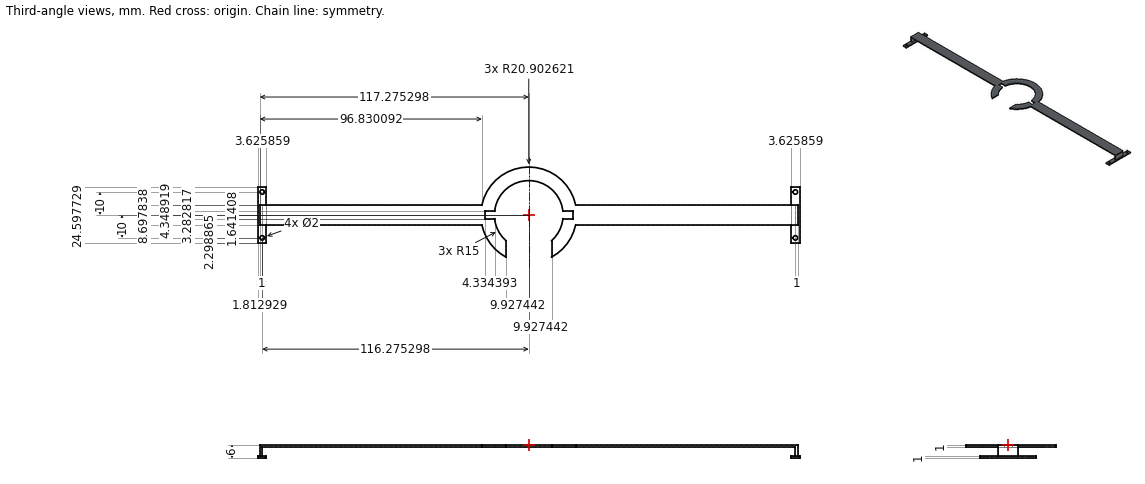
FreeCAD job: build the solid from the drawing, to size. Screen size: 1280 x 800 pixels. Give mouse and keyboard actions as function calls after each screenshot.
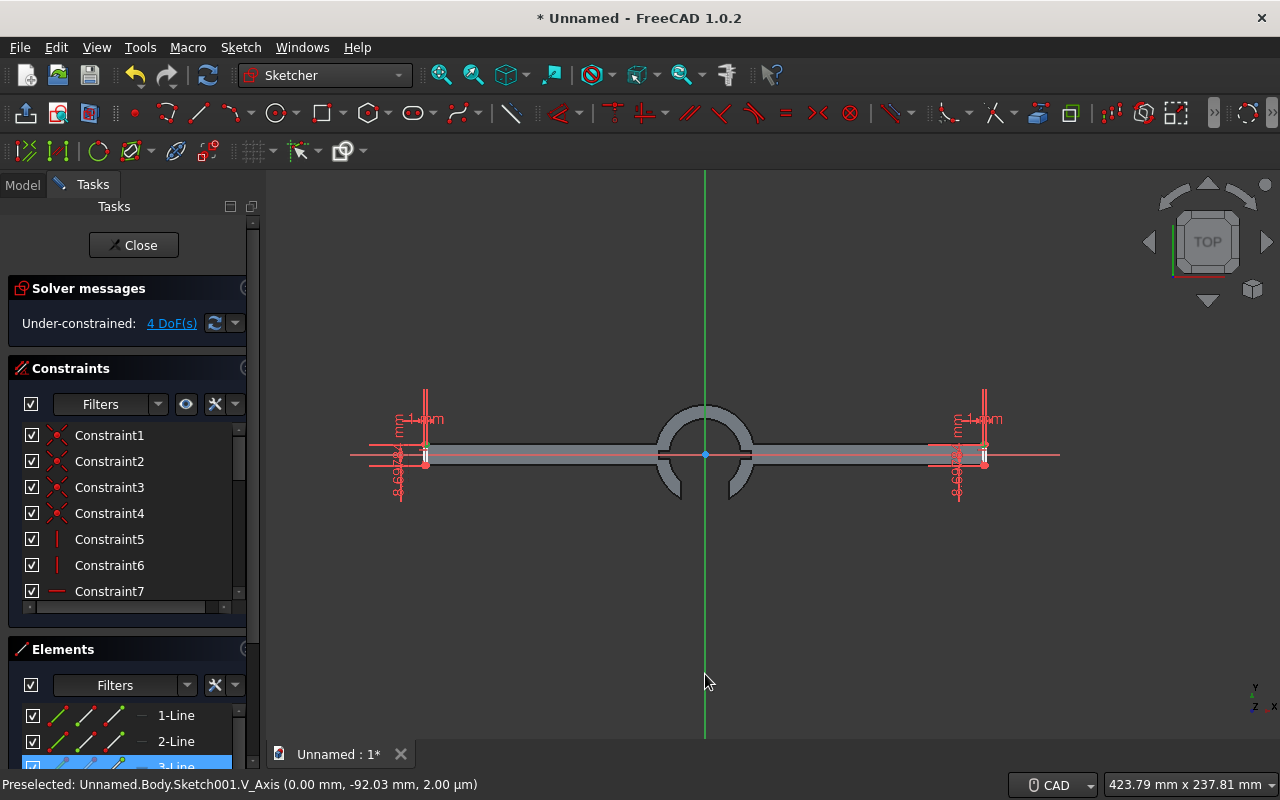
click(818, 114)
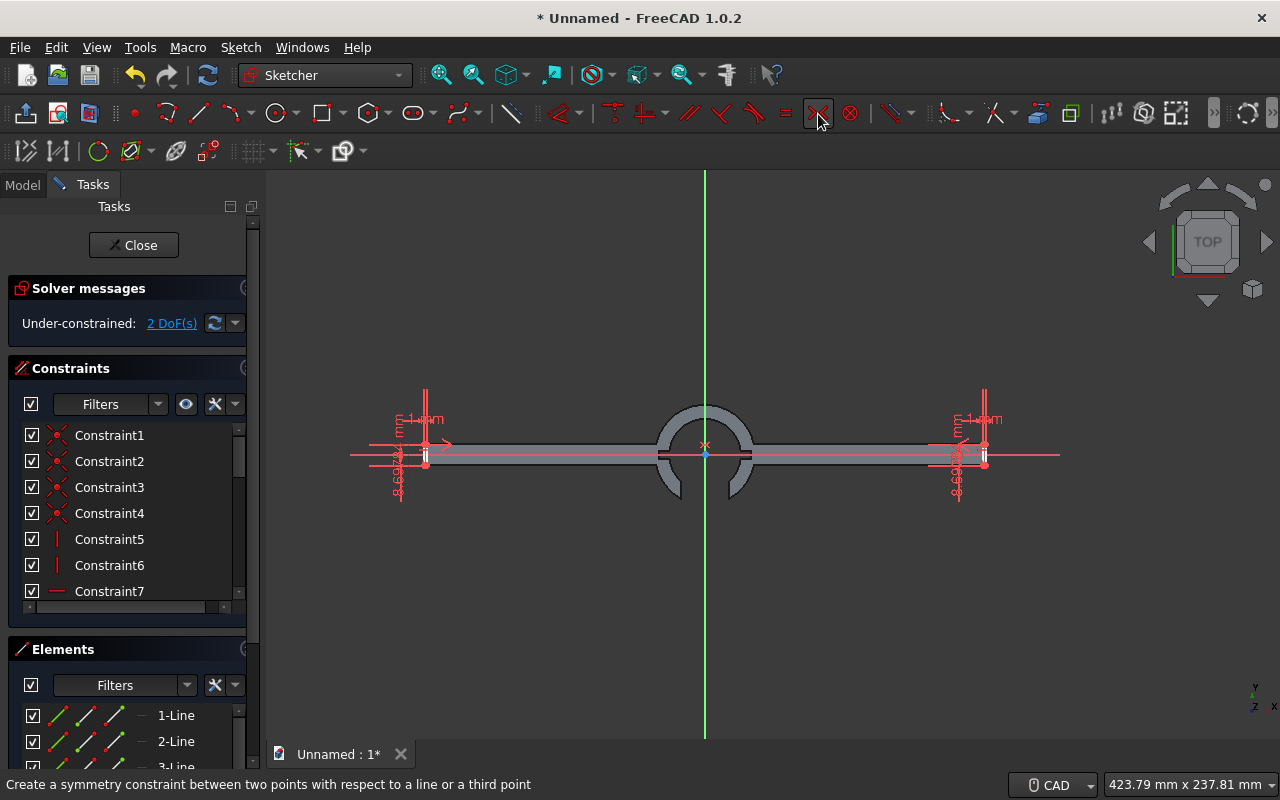
click(558, 114)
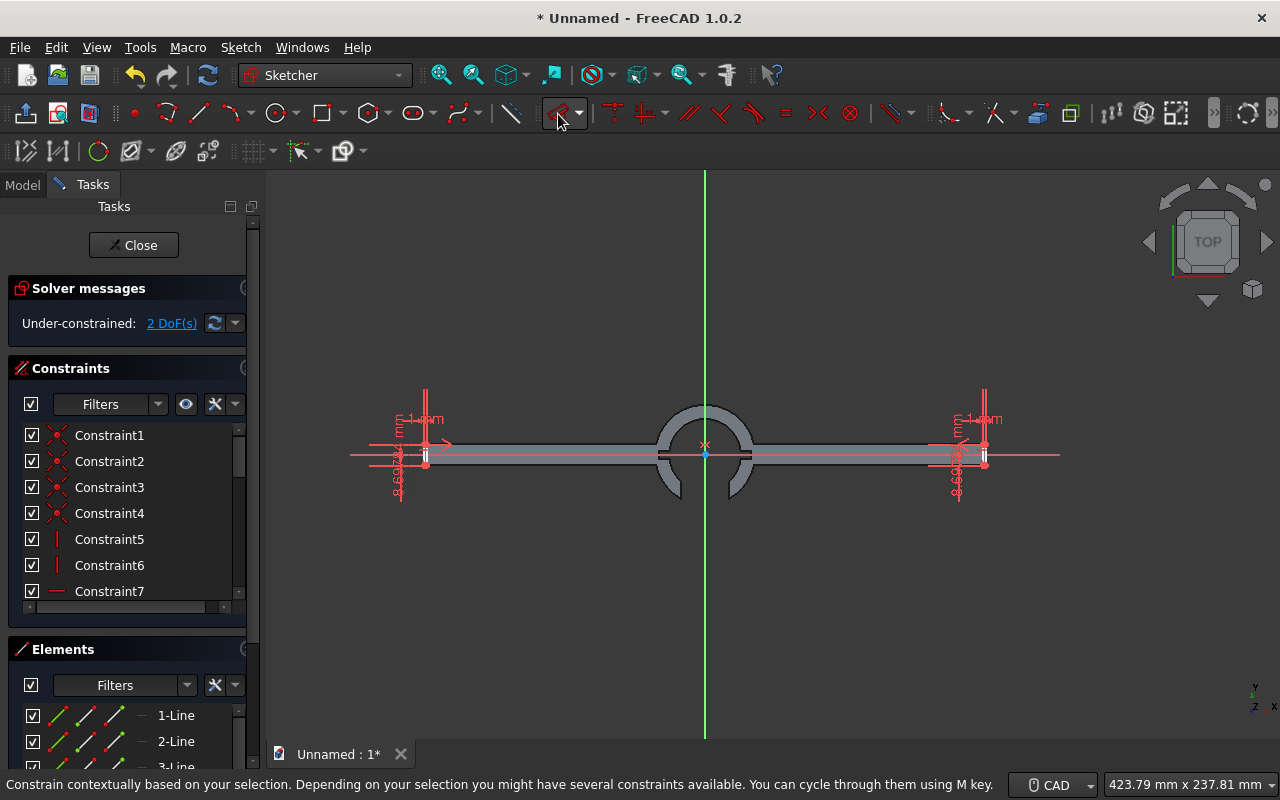
scroll(424, 445, up, 9)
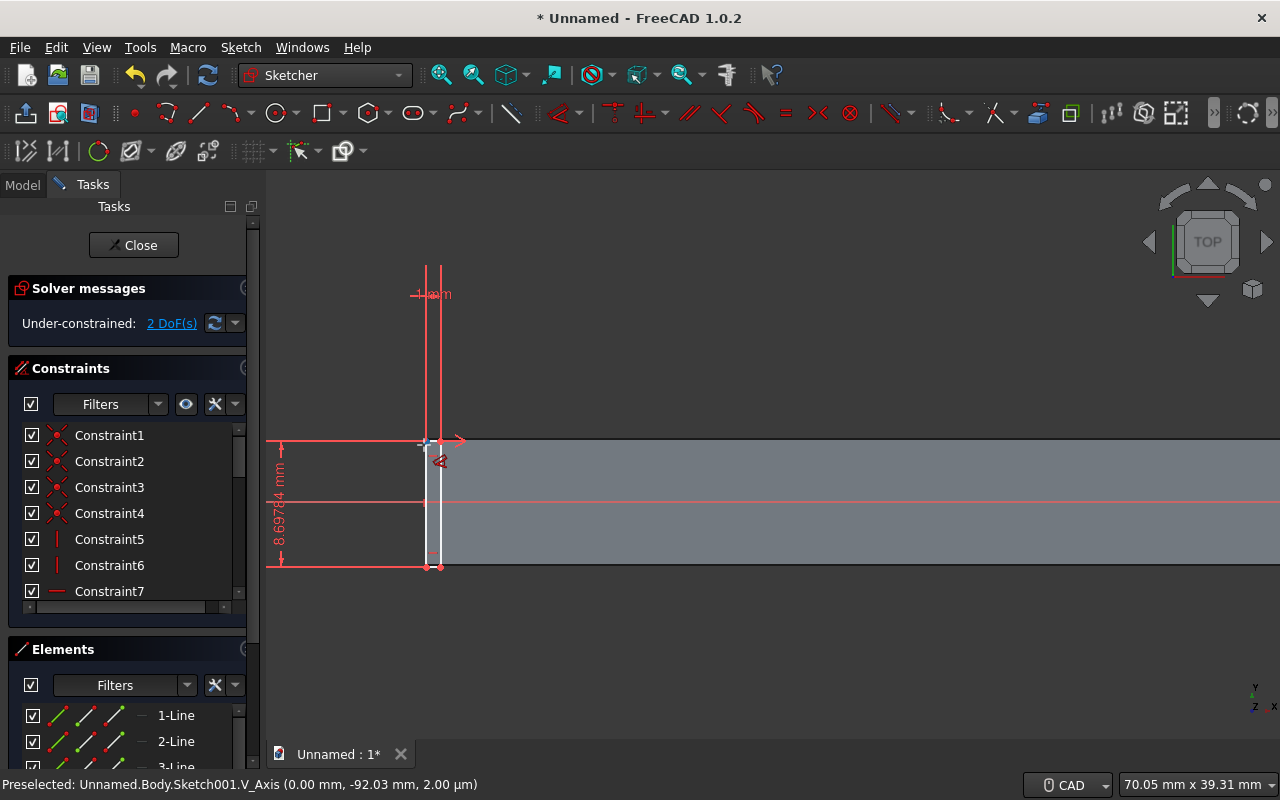
click(426, 441)
click(392, 471)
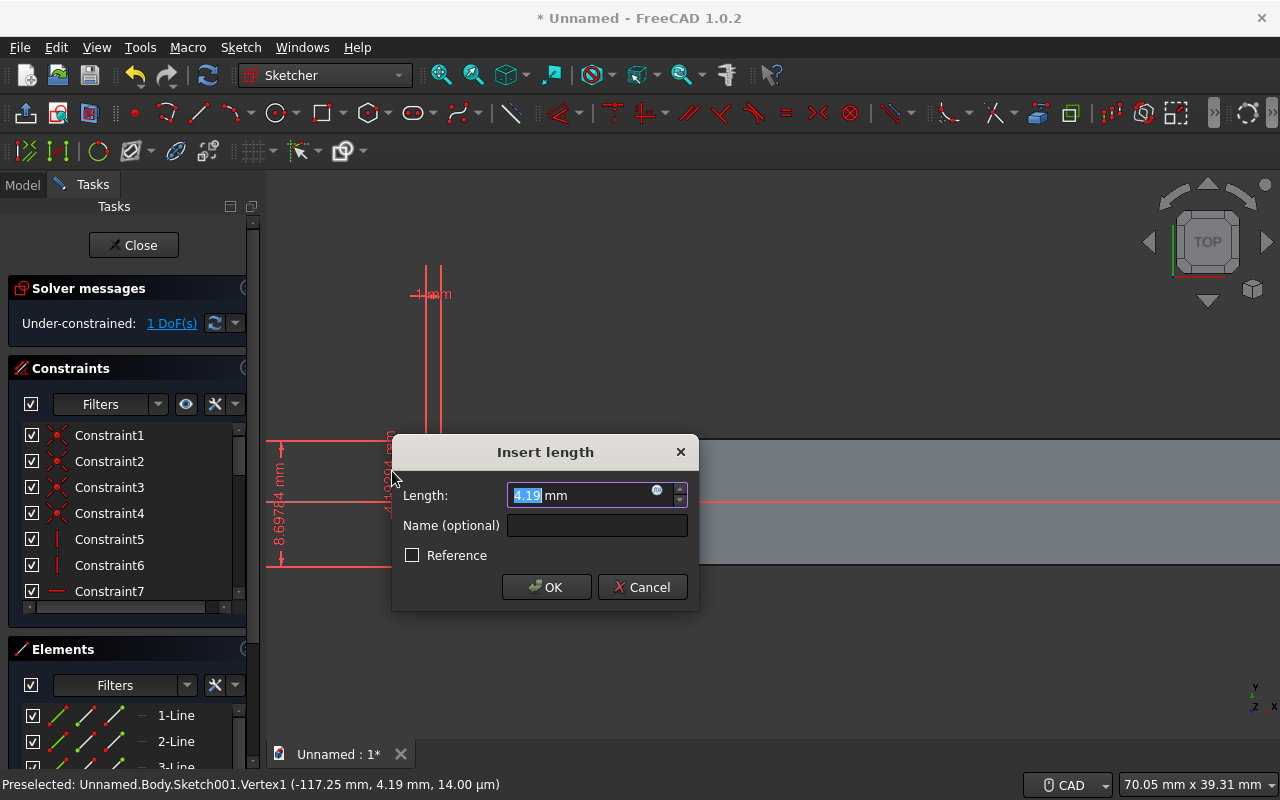
text(4.348919)
key(Return)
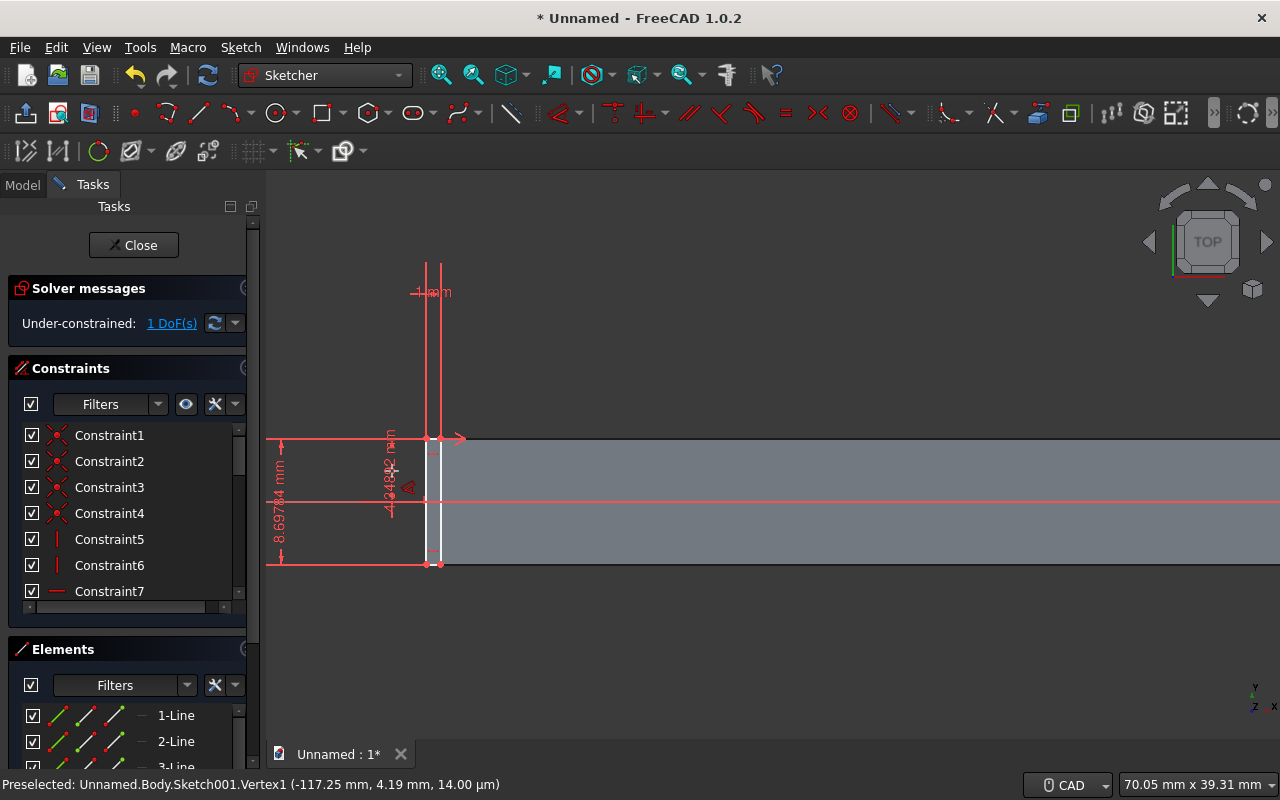
click(426, 439)
click(771, 405)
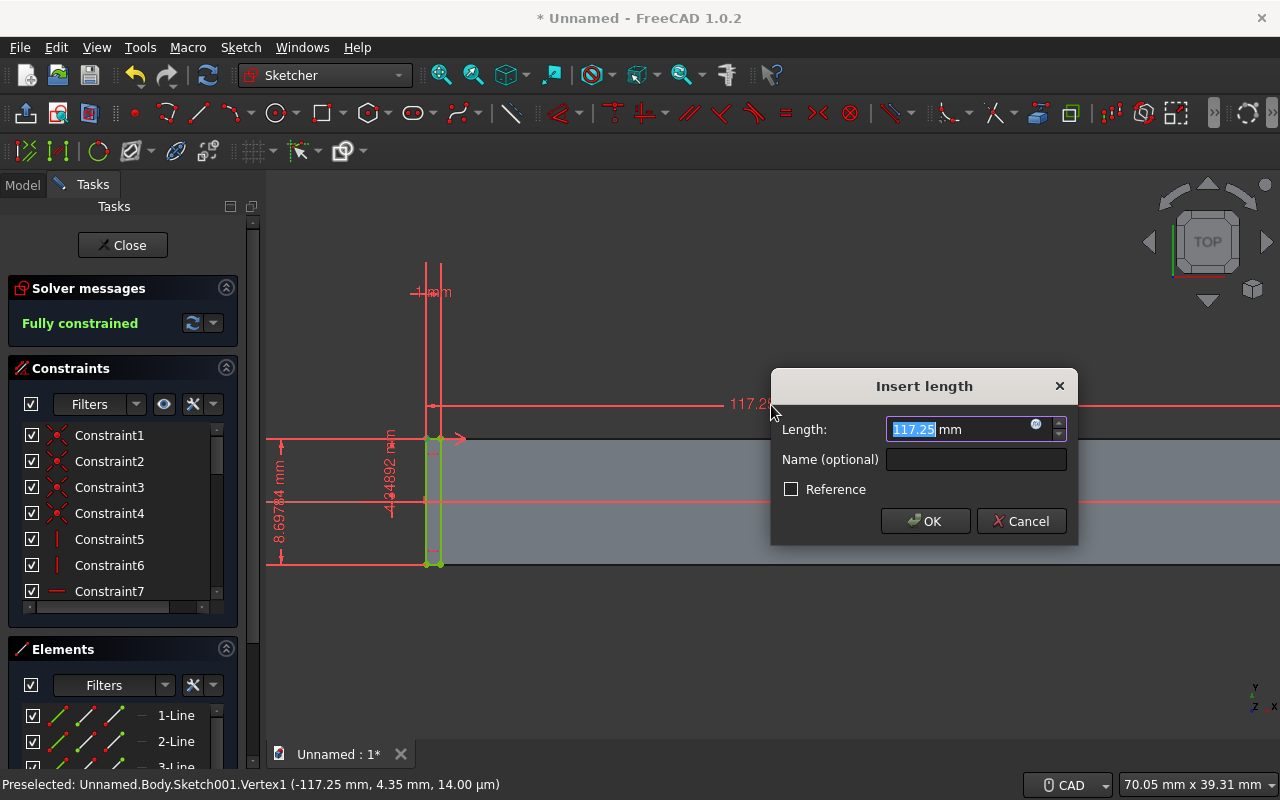
text(117.275298)
key(Return)
key(Escape)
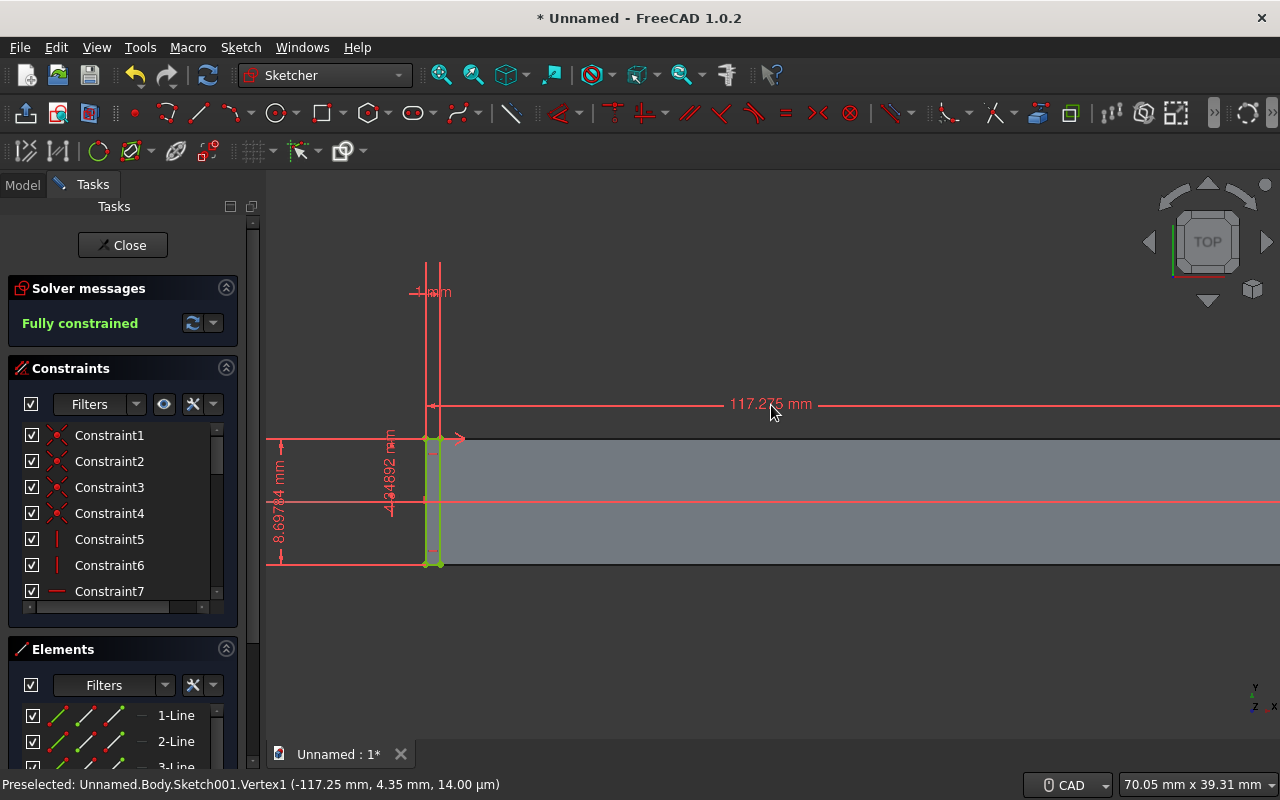
click(123, 245)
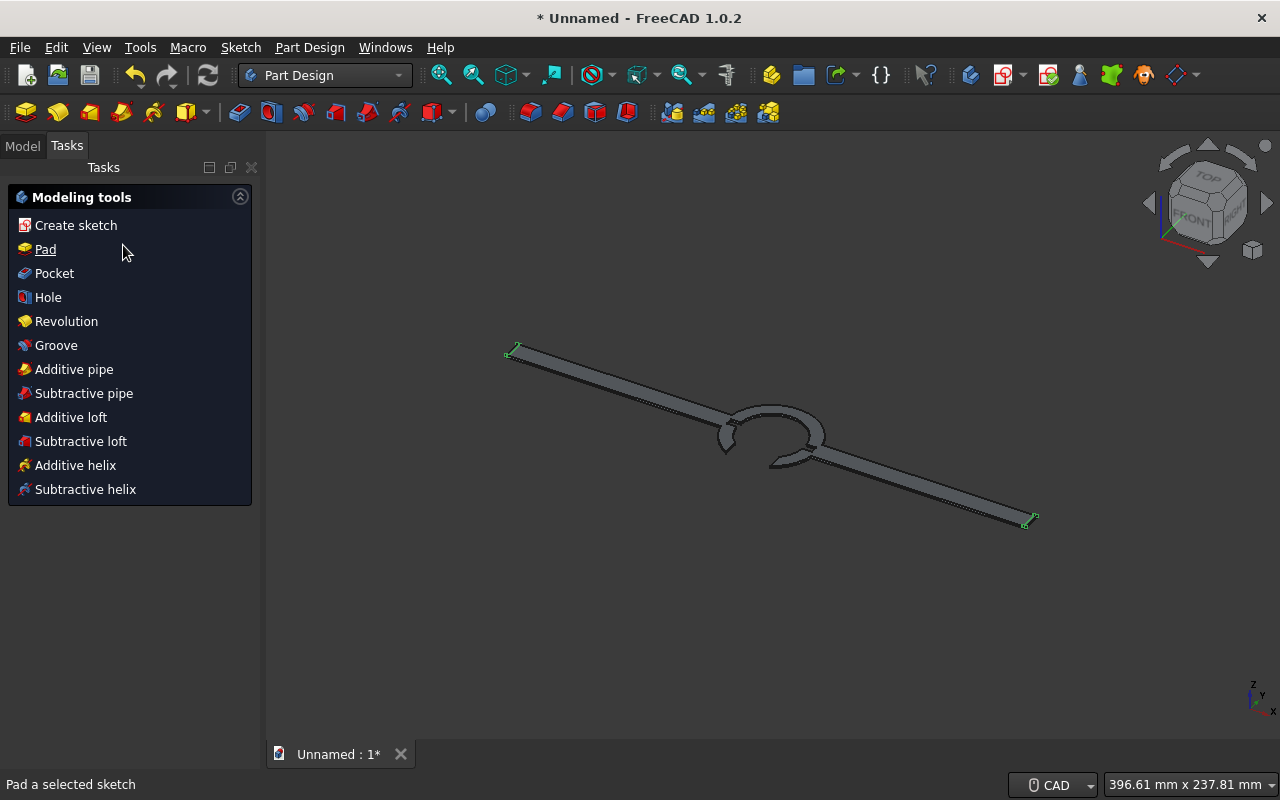
click(26, 112)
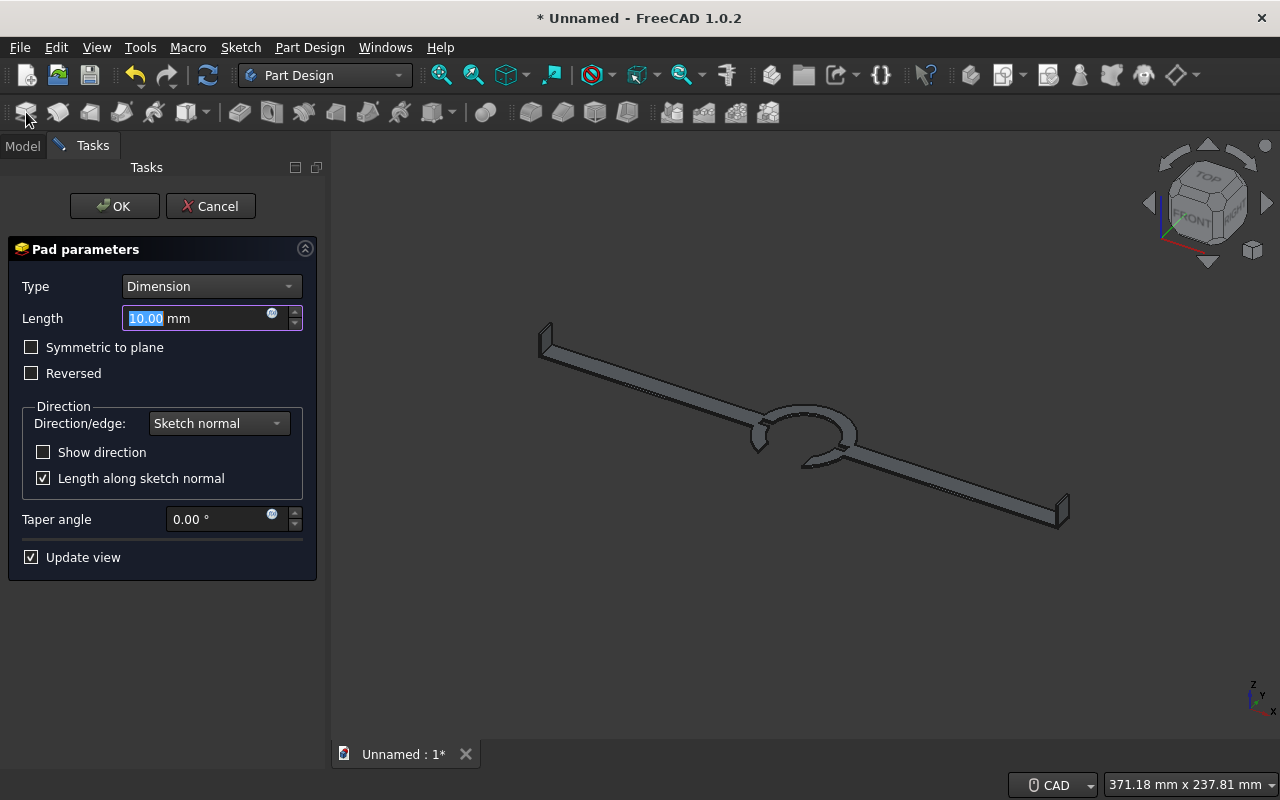
text(6)
key(Tab)